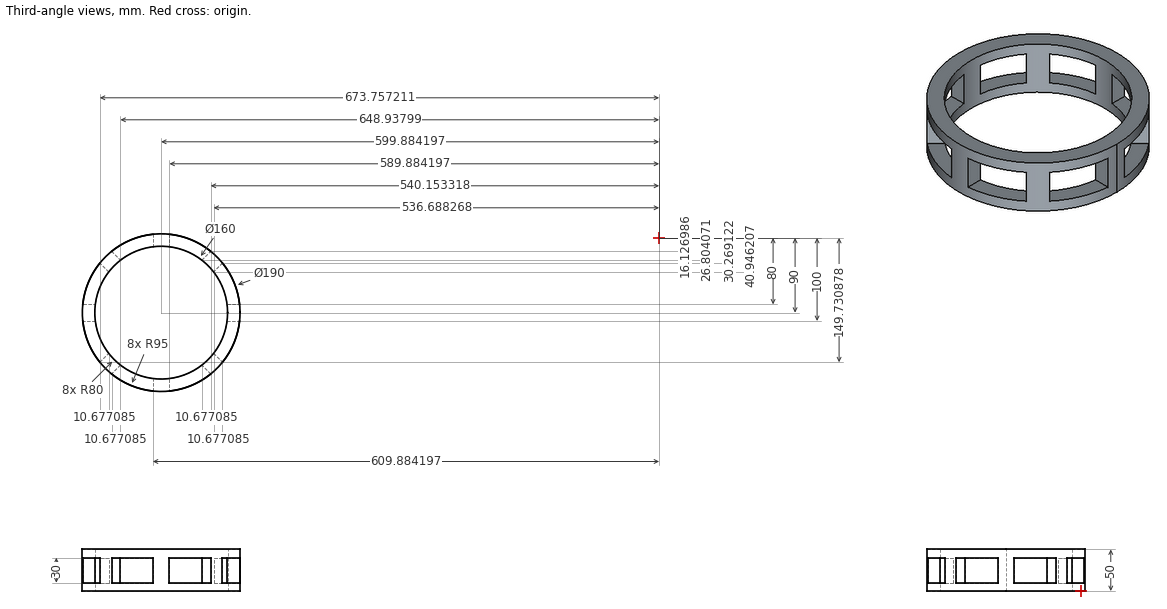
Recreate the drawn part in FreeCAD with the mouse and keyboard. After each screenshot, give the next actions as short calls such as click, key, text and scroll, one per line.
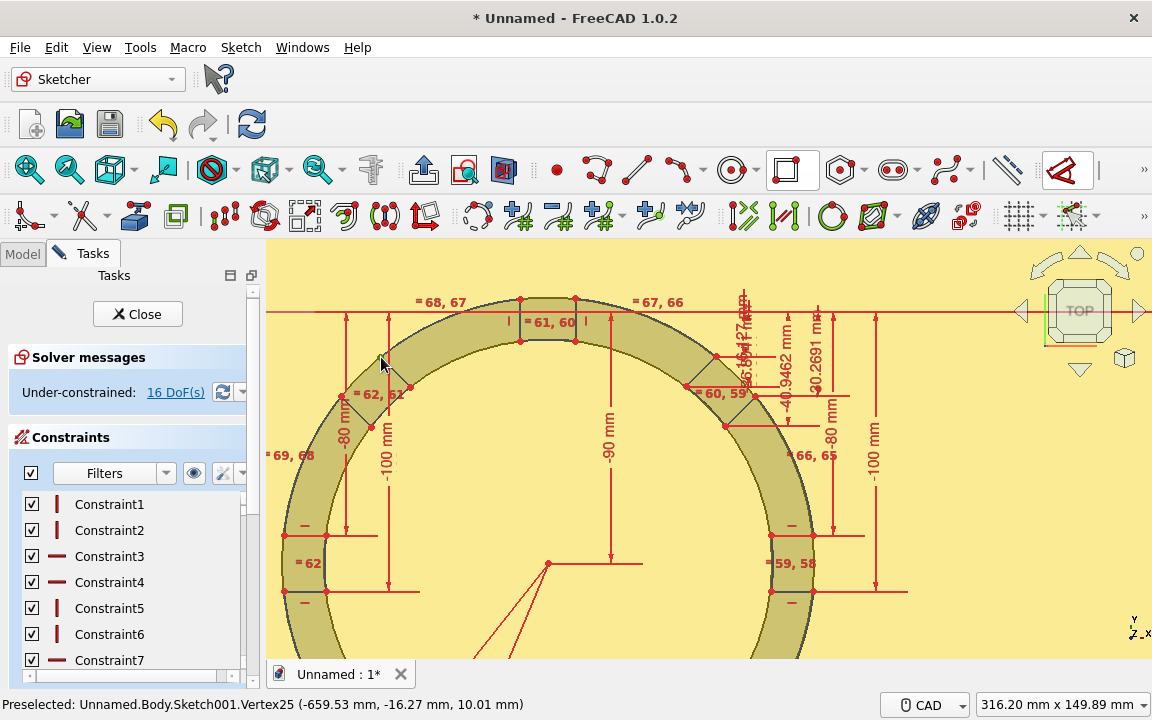
click(1088, 170)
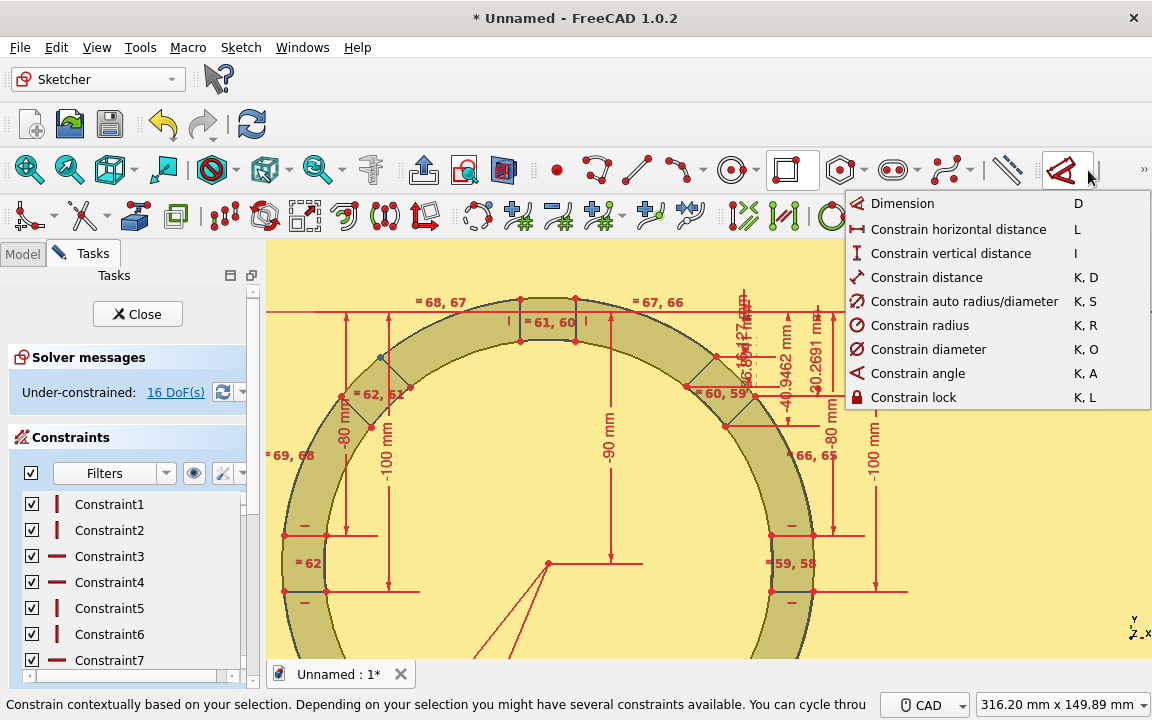
click(998, 253)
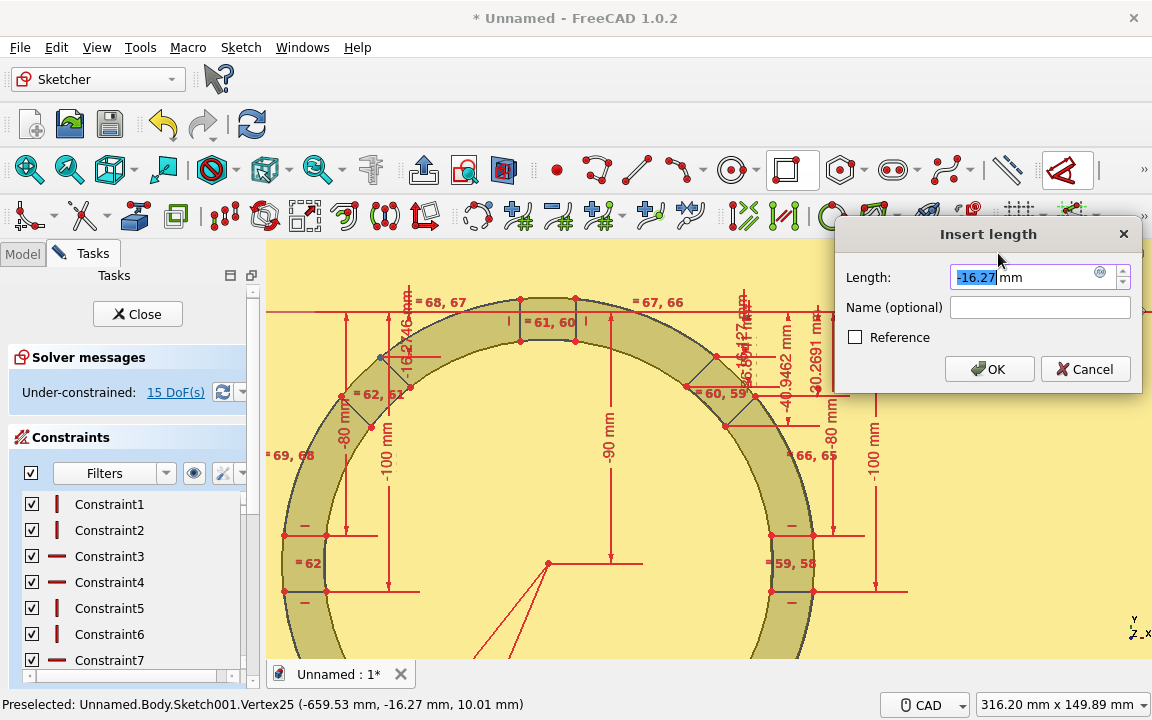
text(-16.126986)
key(Return)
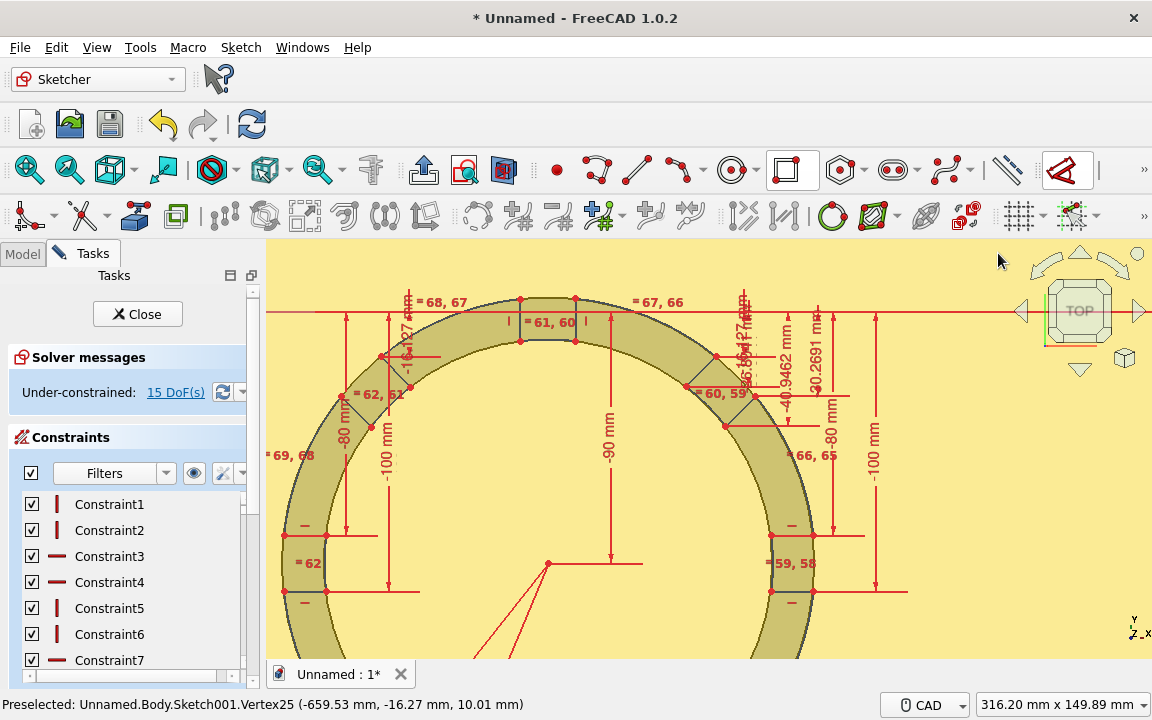
click(410, 387)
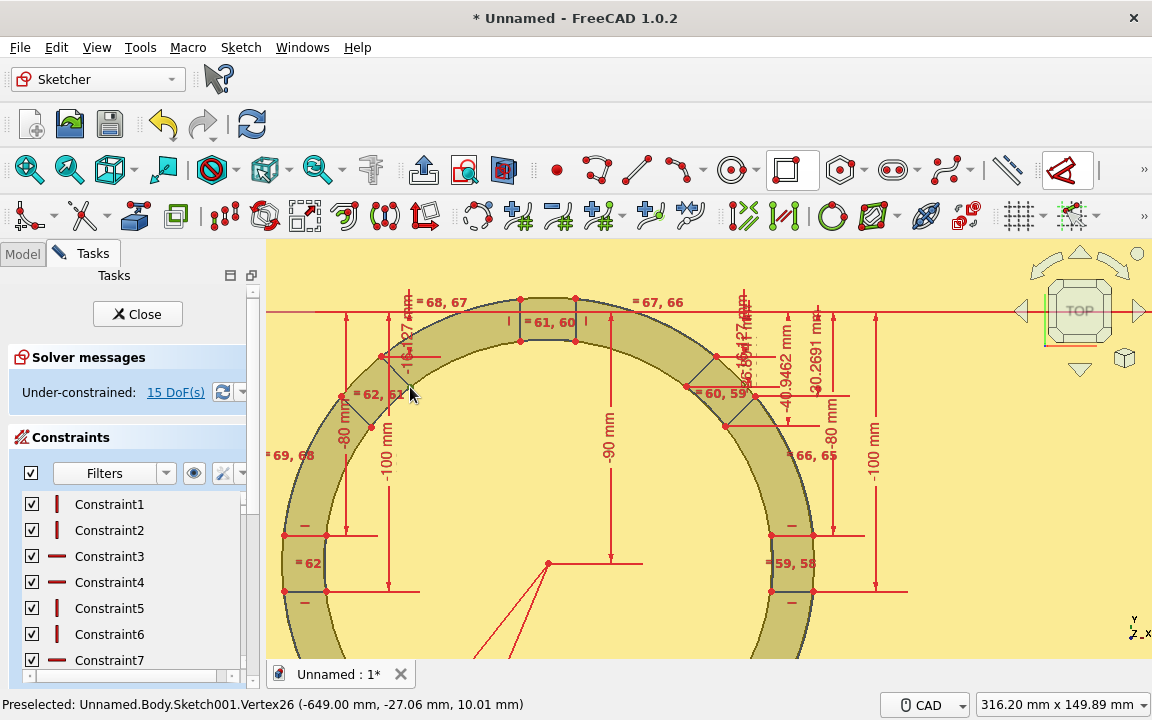
key(l)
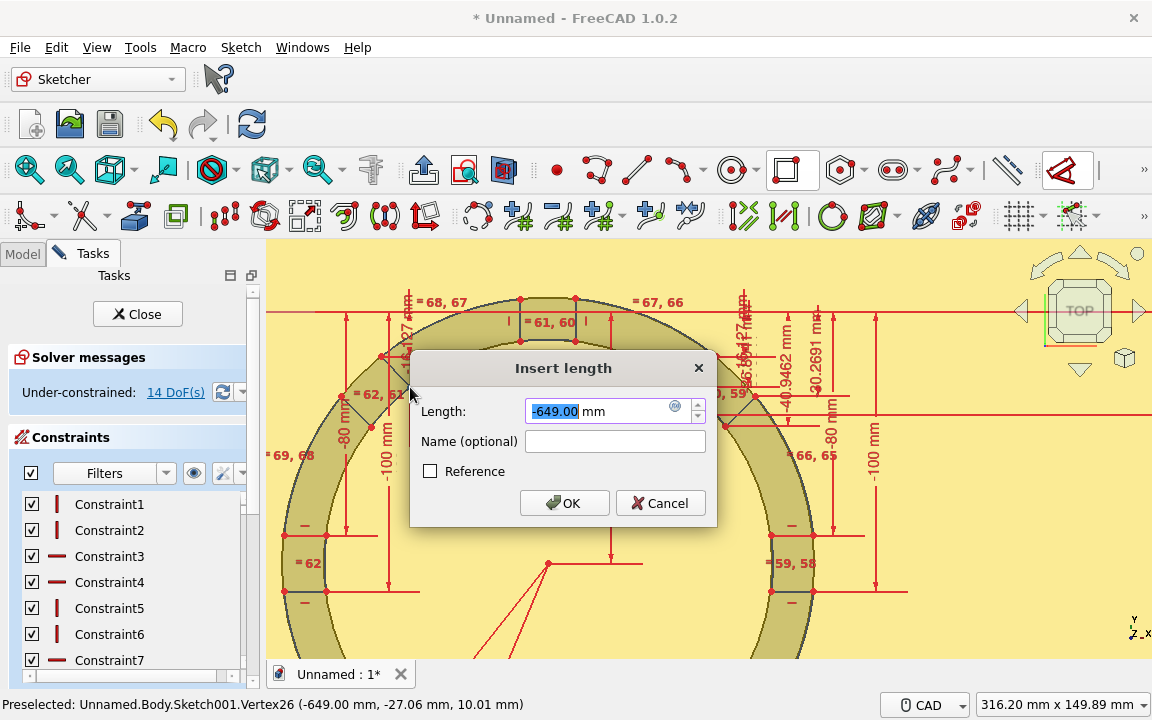
text(-648.93799)
key(Return)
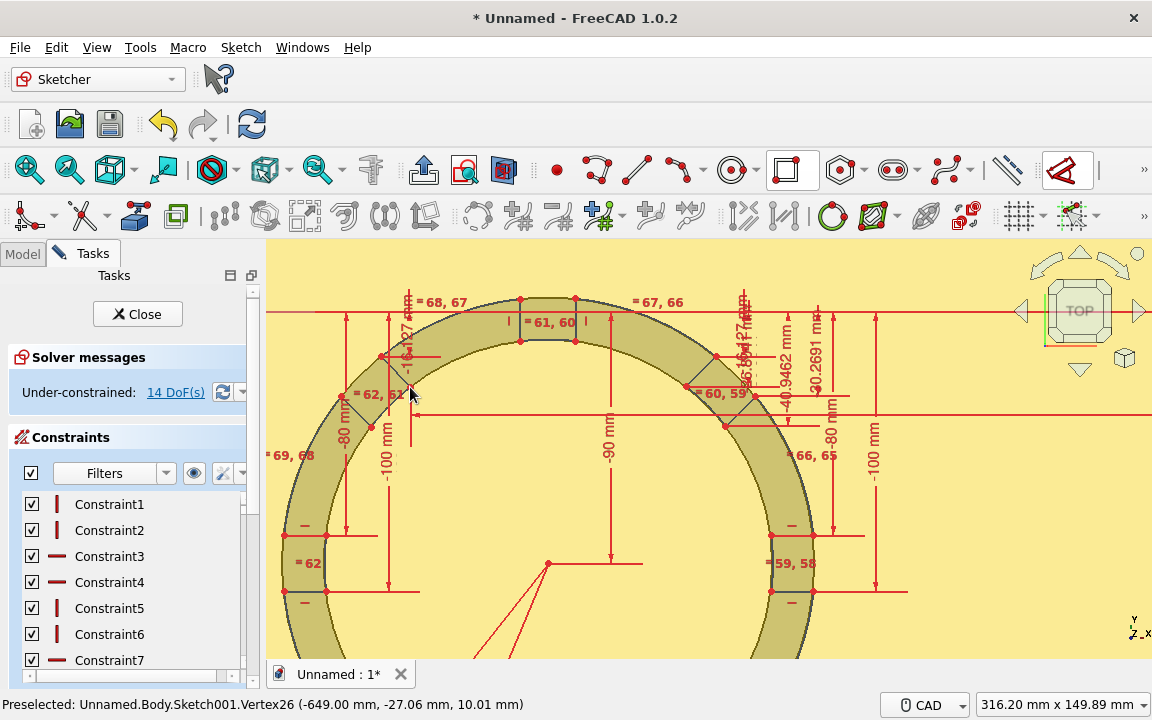
click(371, 427)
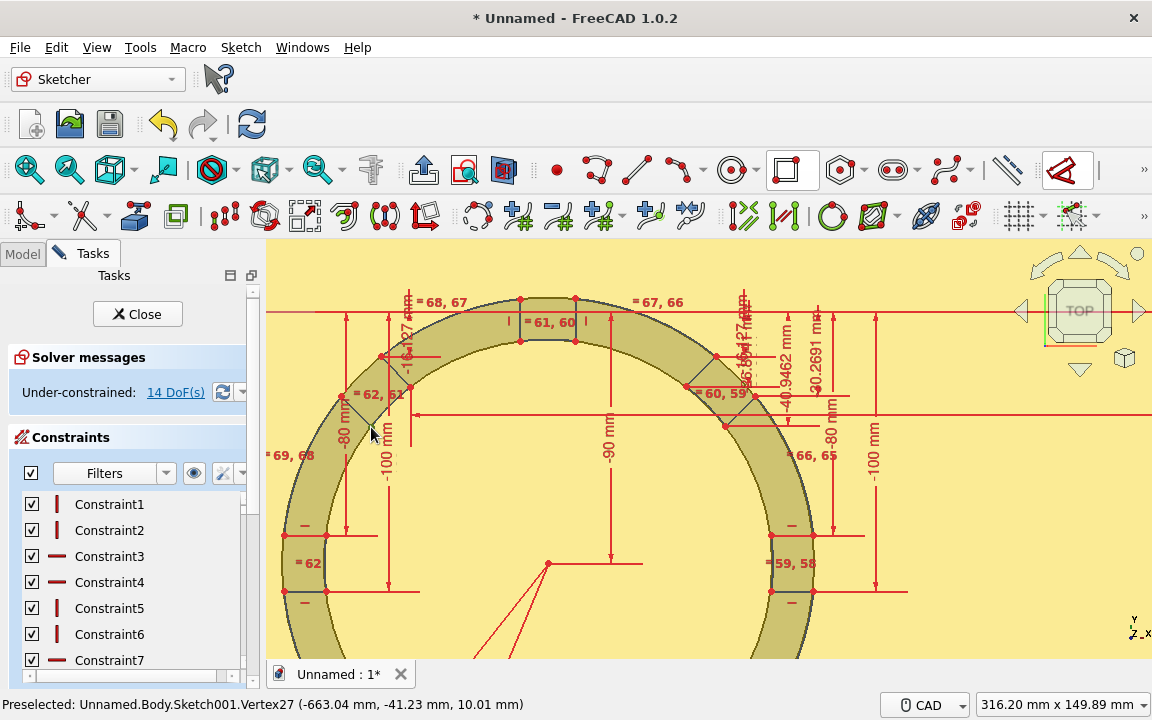
key(i)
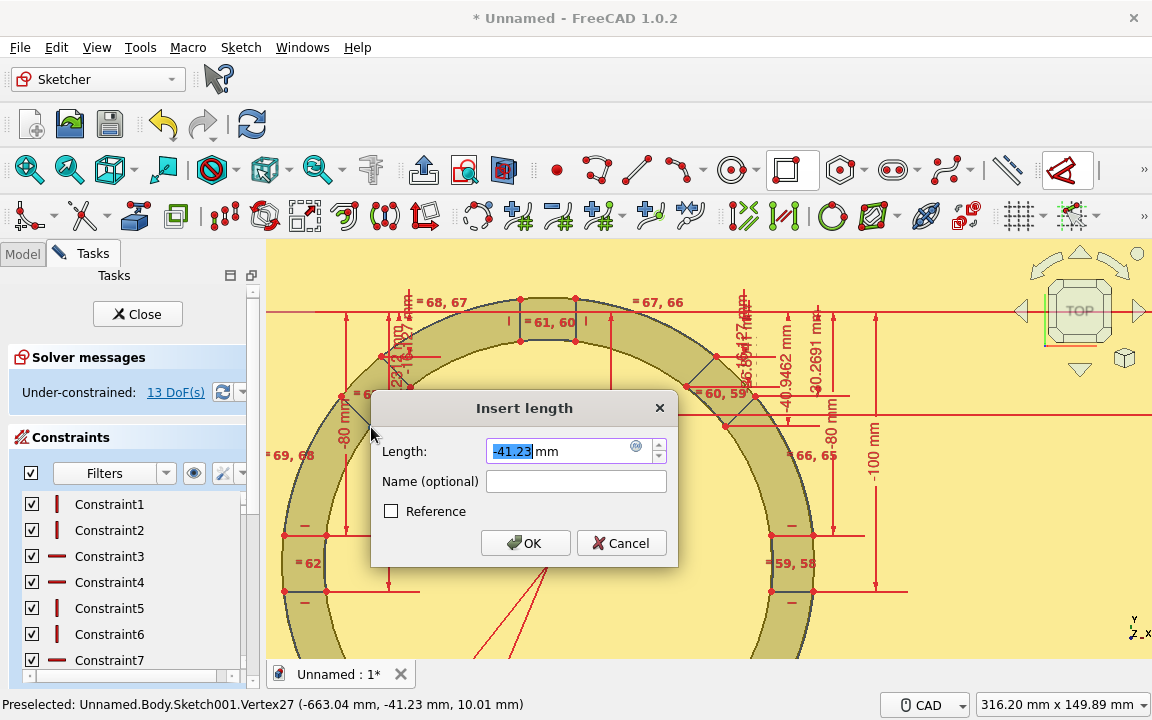
text(-40.946207)
key(Return)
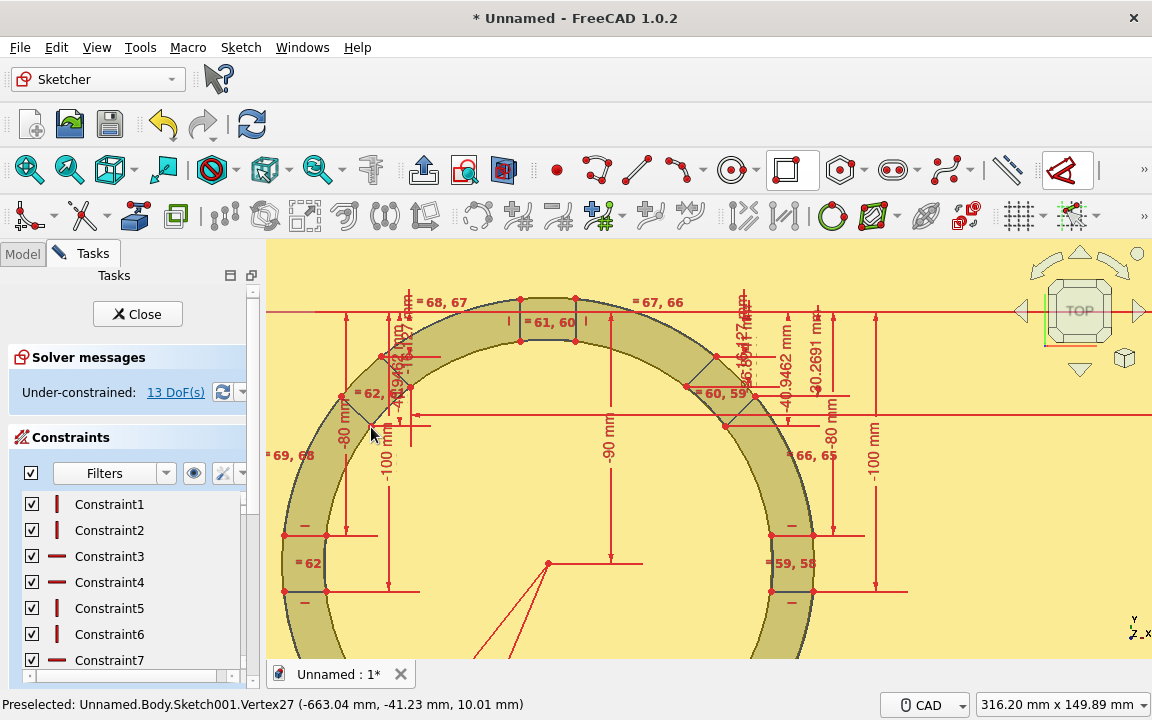
click(341, 397)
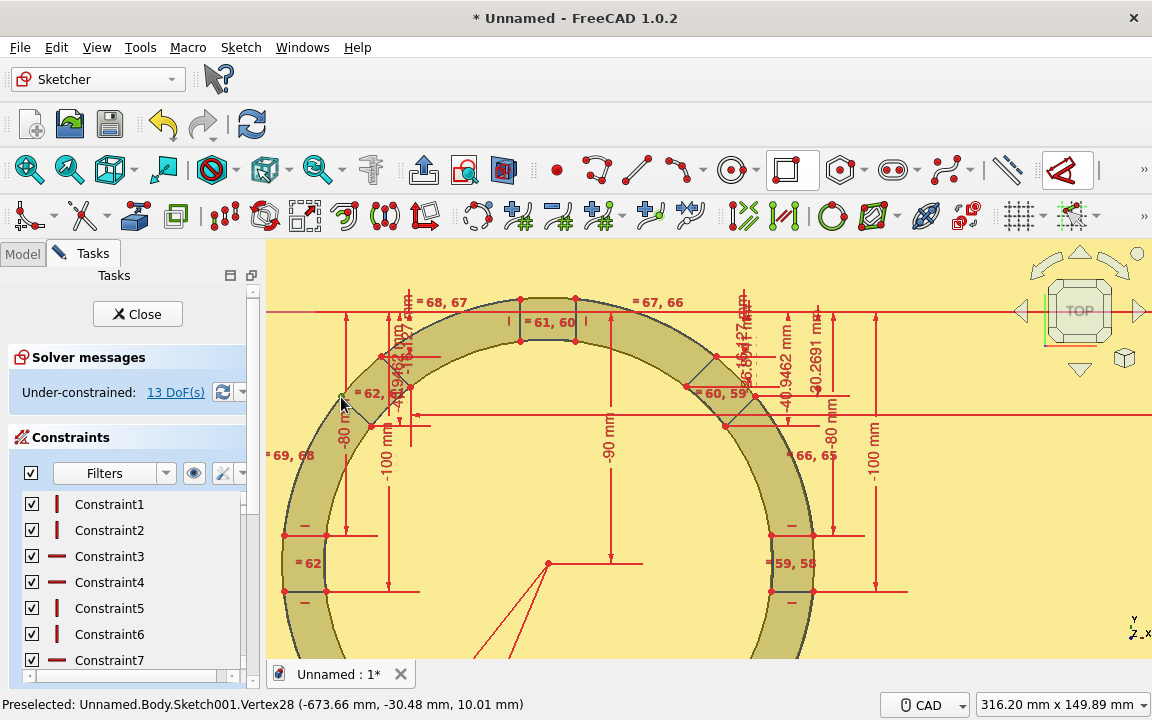
key(i)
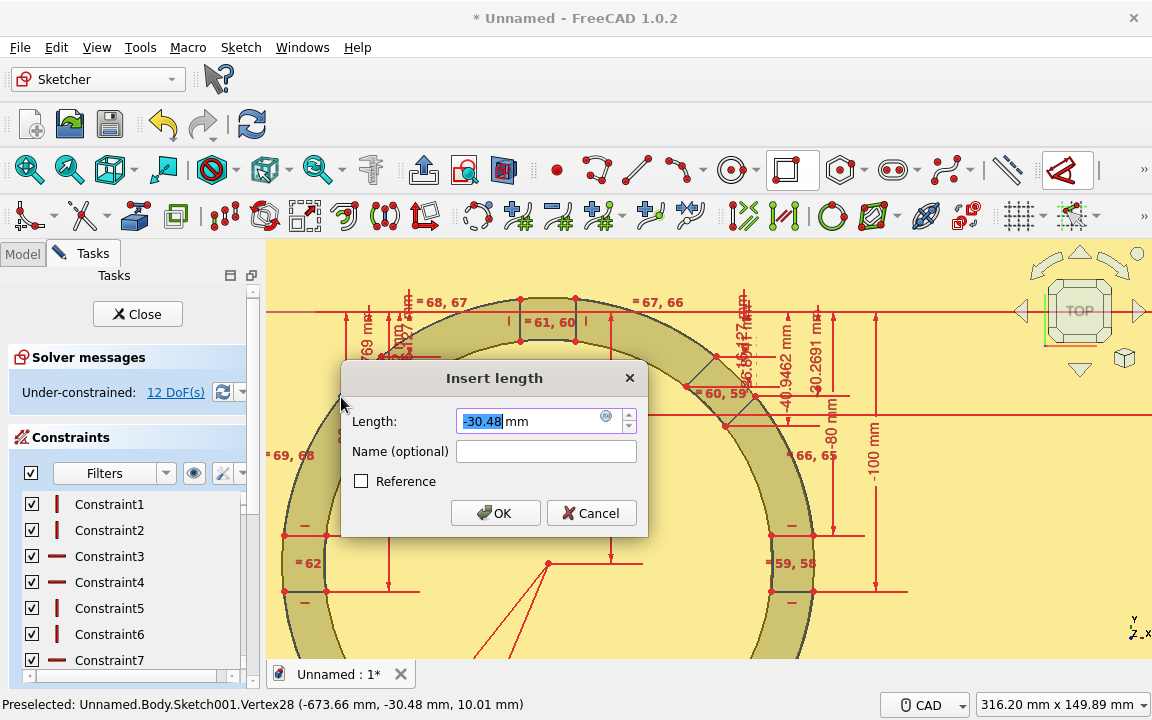
text(-30.269122)
key(Return)